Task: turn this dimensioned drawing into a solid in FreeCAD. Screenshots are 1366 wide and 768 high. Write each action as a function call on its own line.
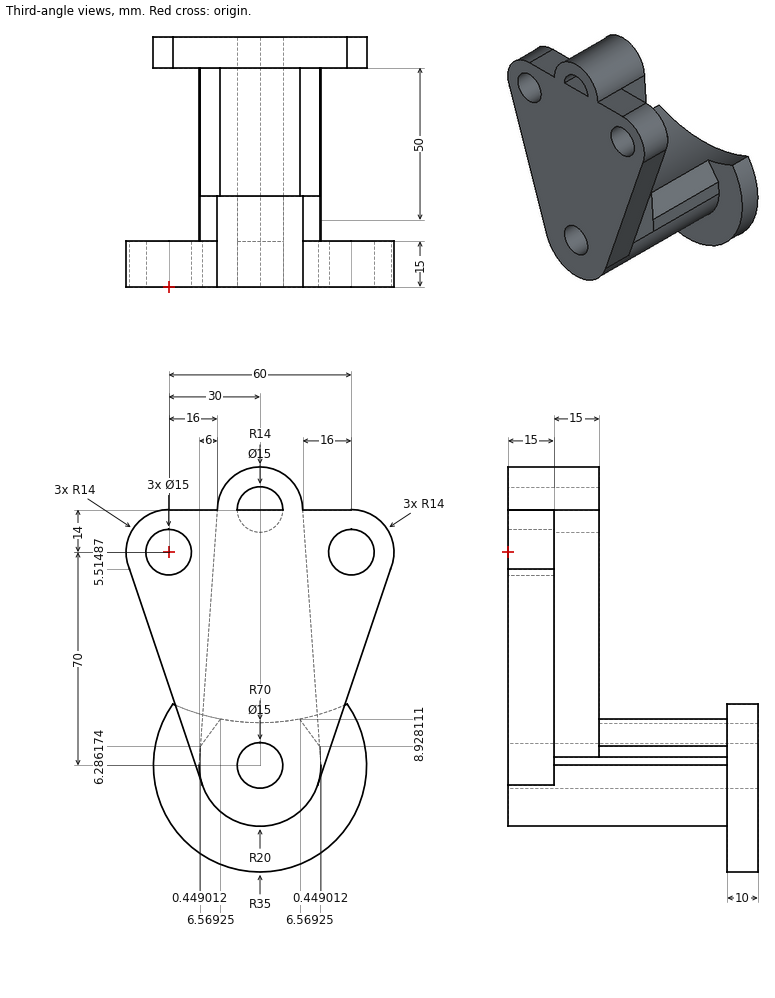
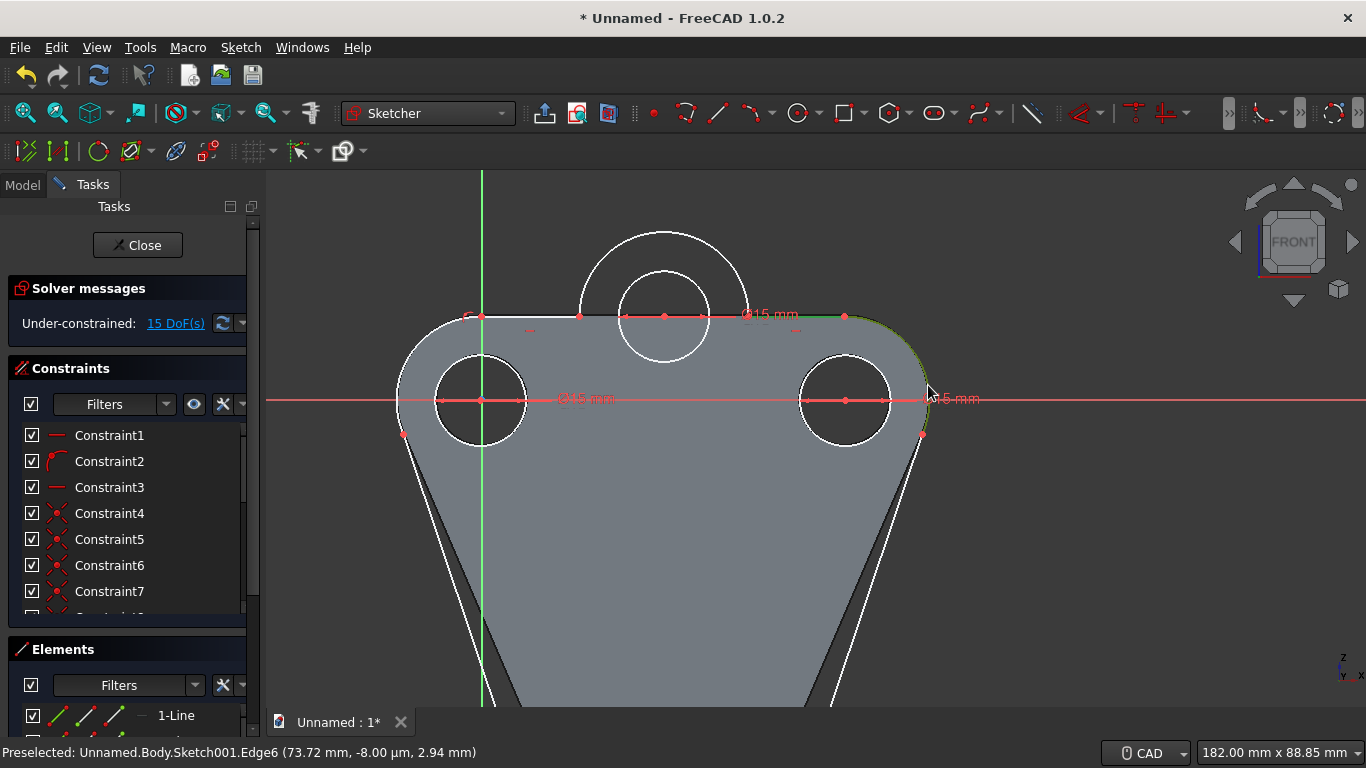
key(t)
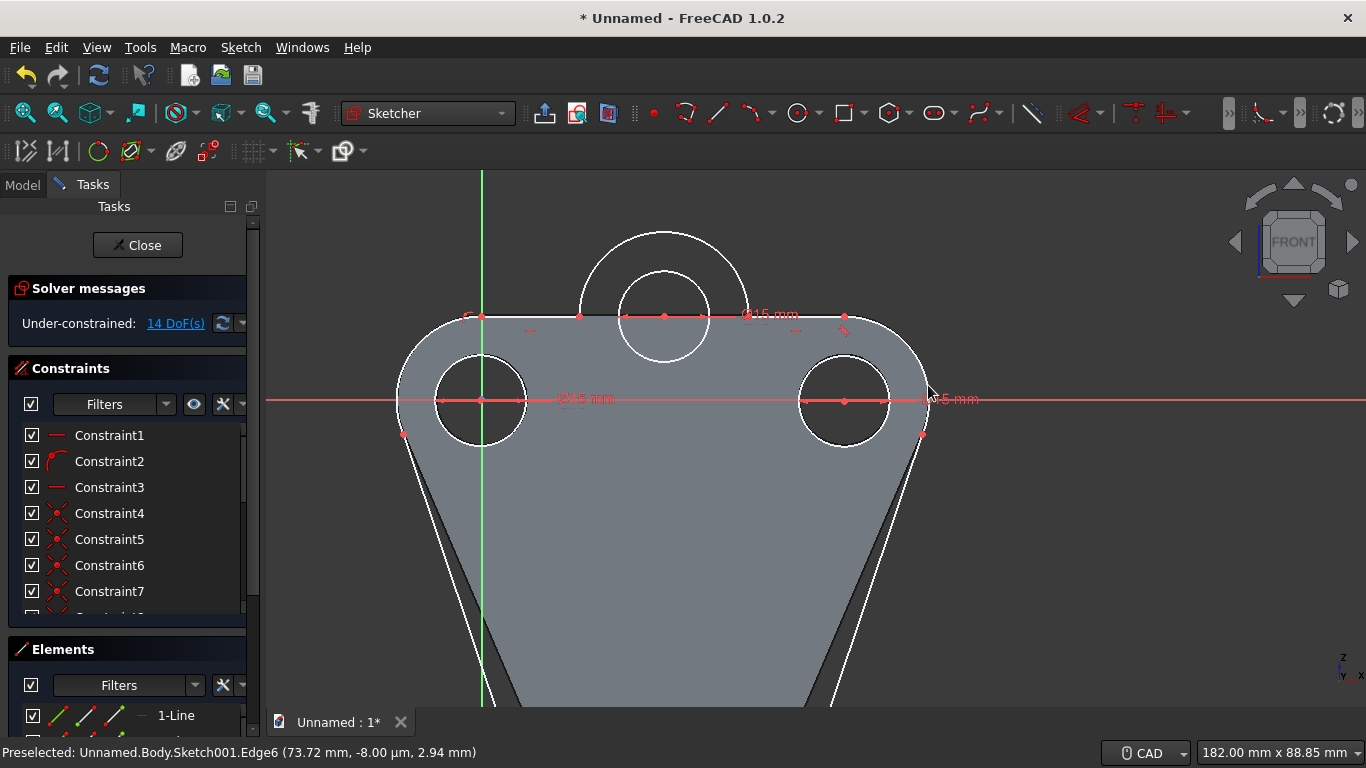
click(550, 317)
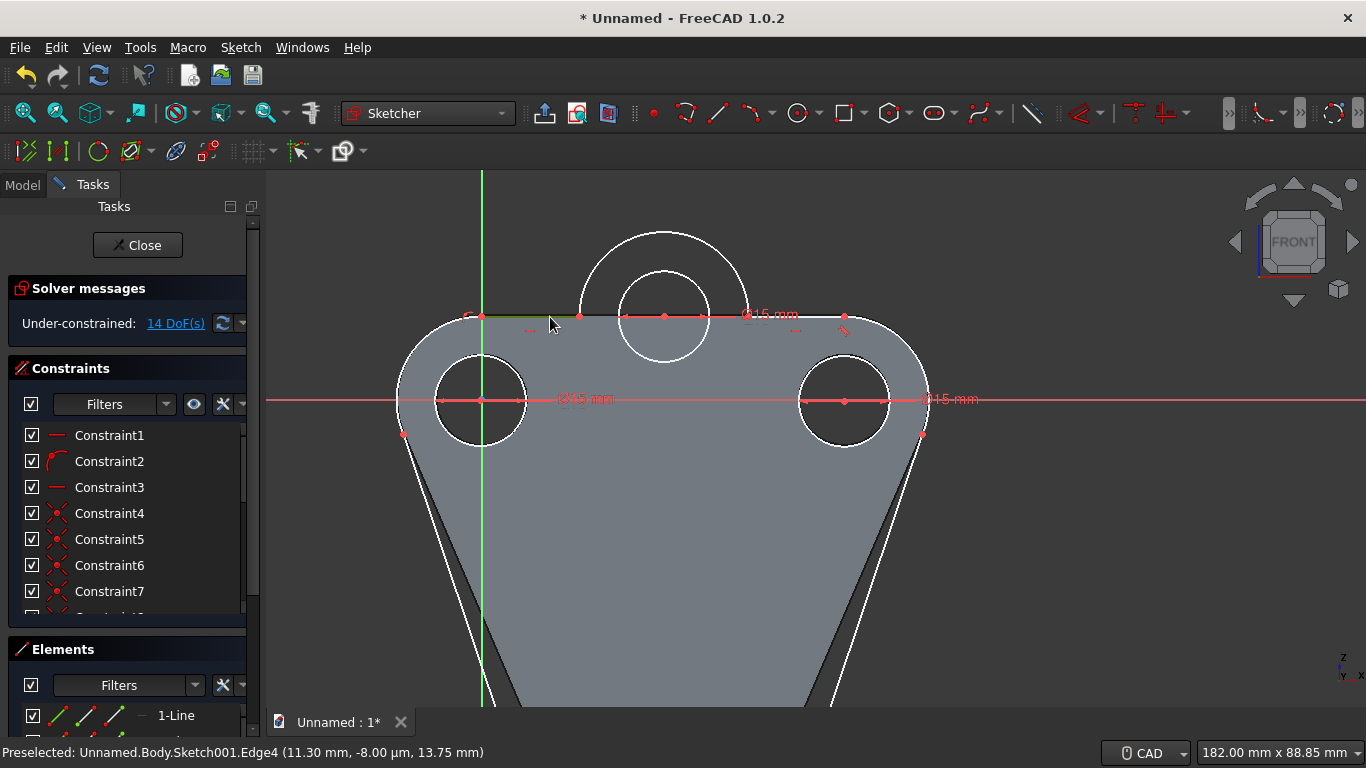
click(434, 331)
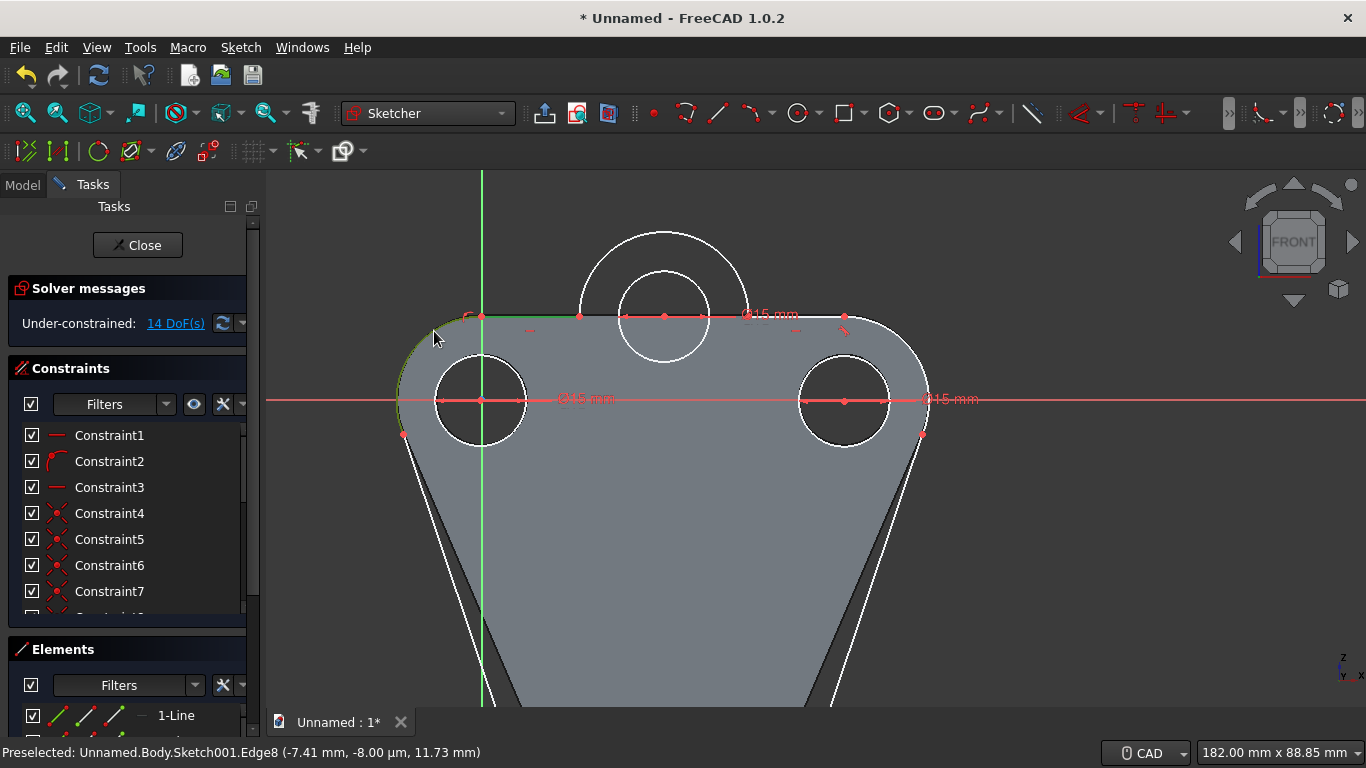
key(t)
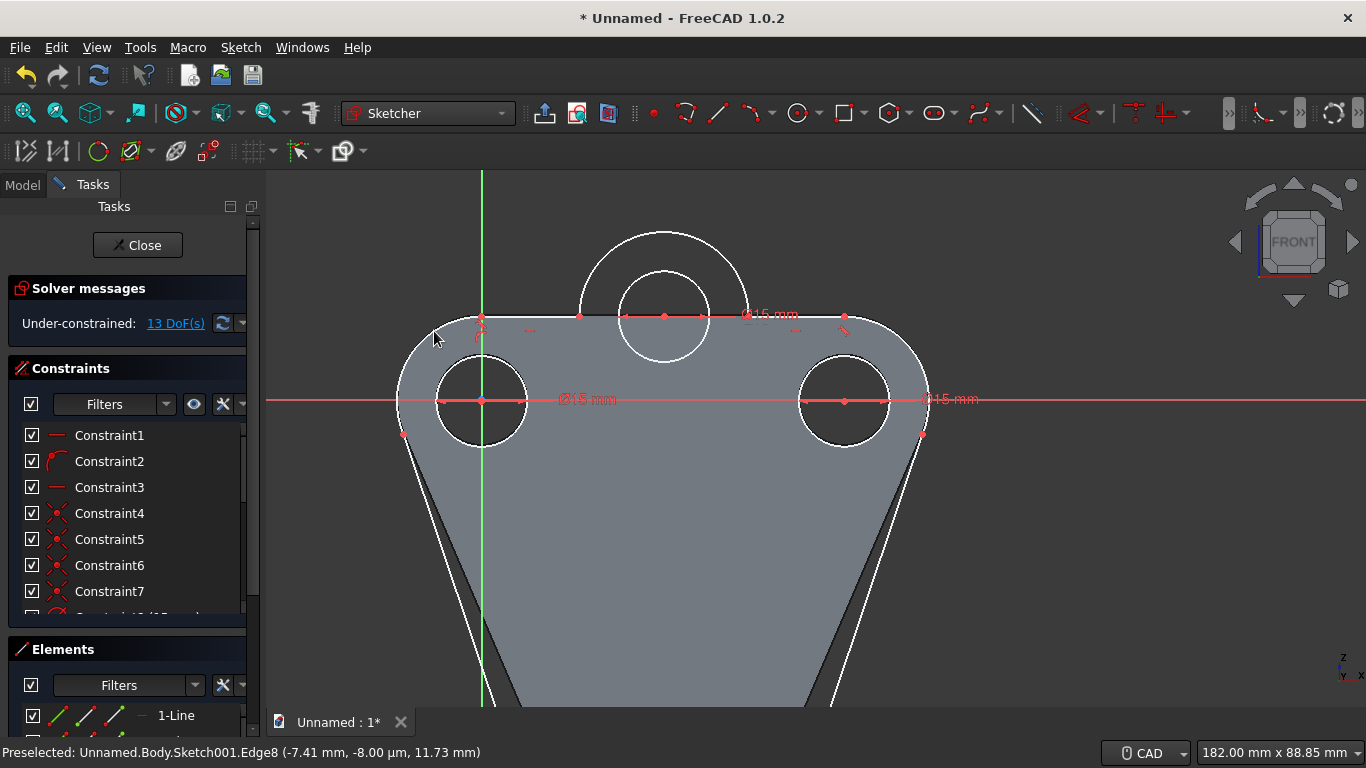
click(928, 385)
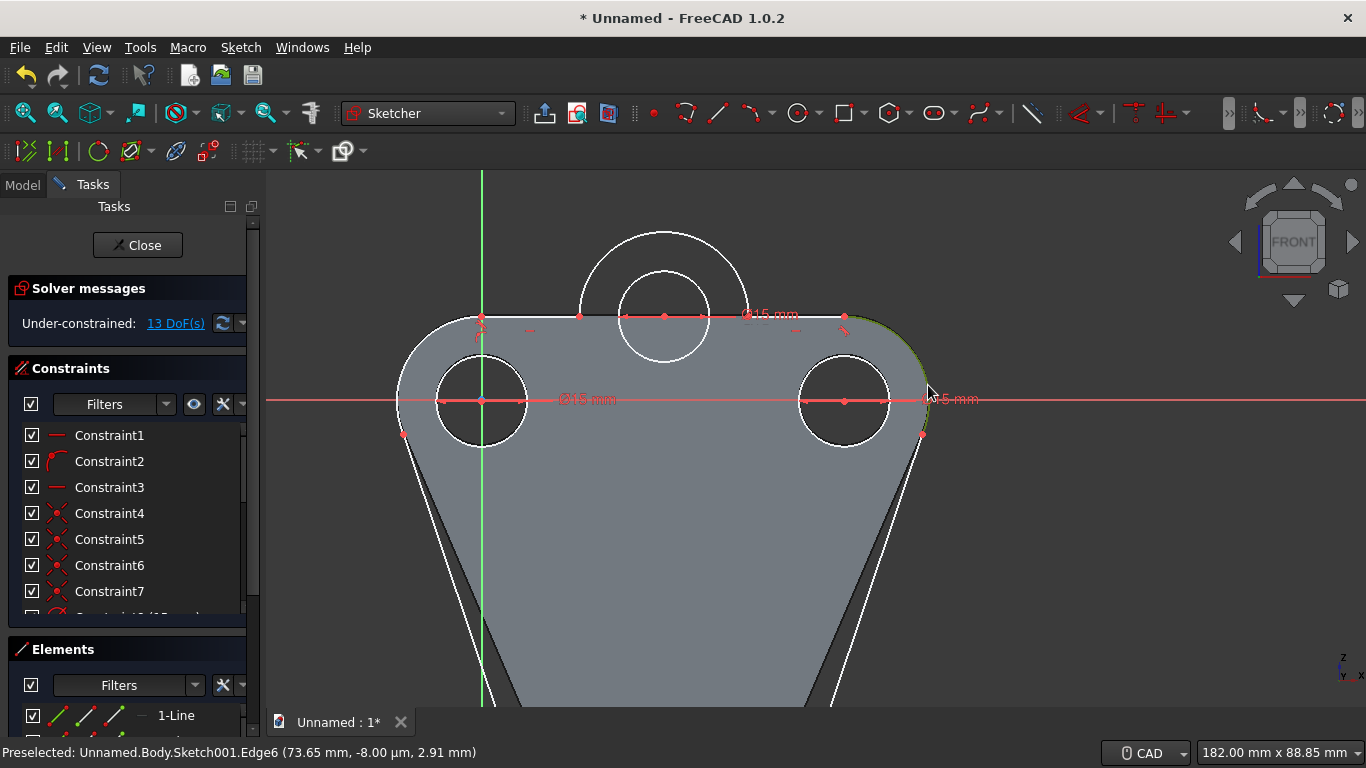
click(714, 248)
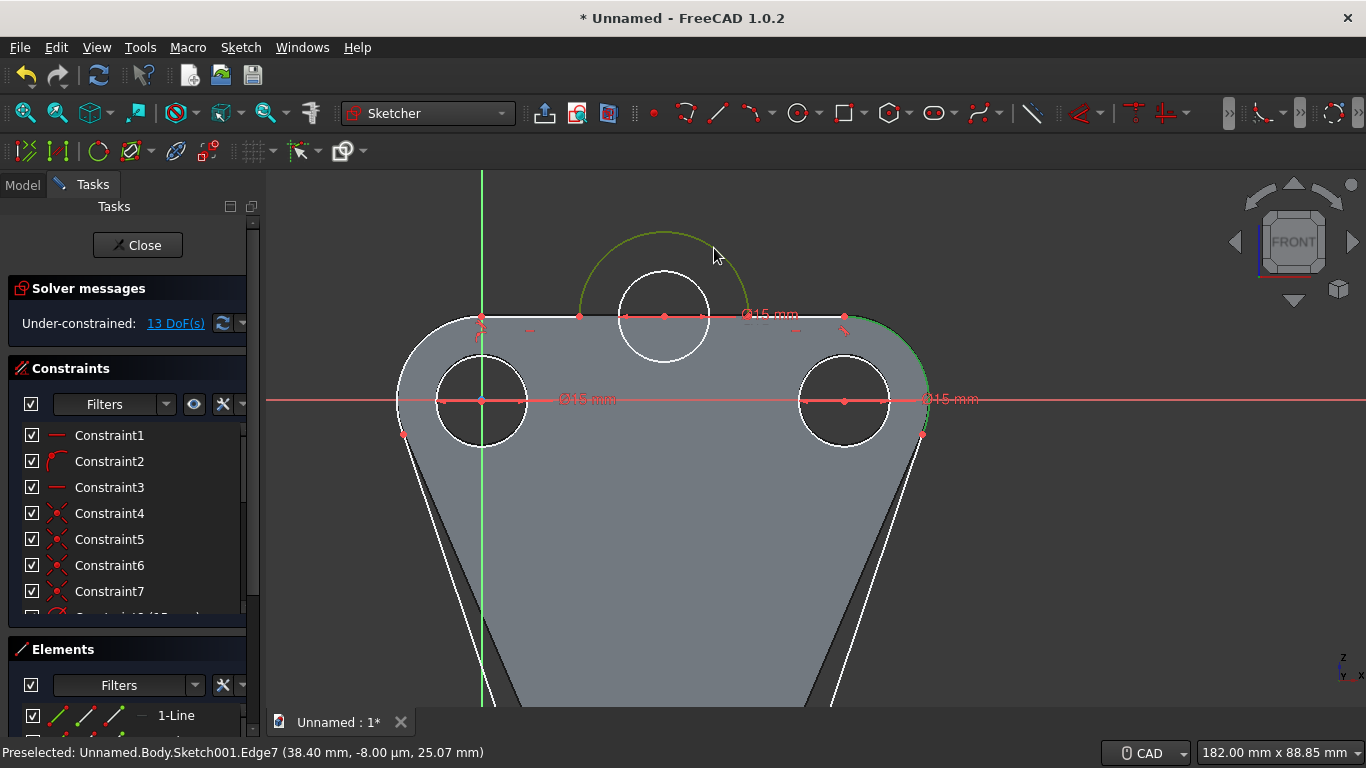
click(434, 331)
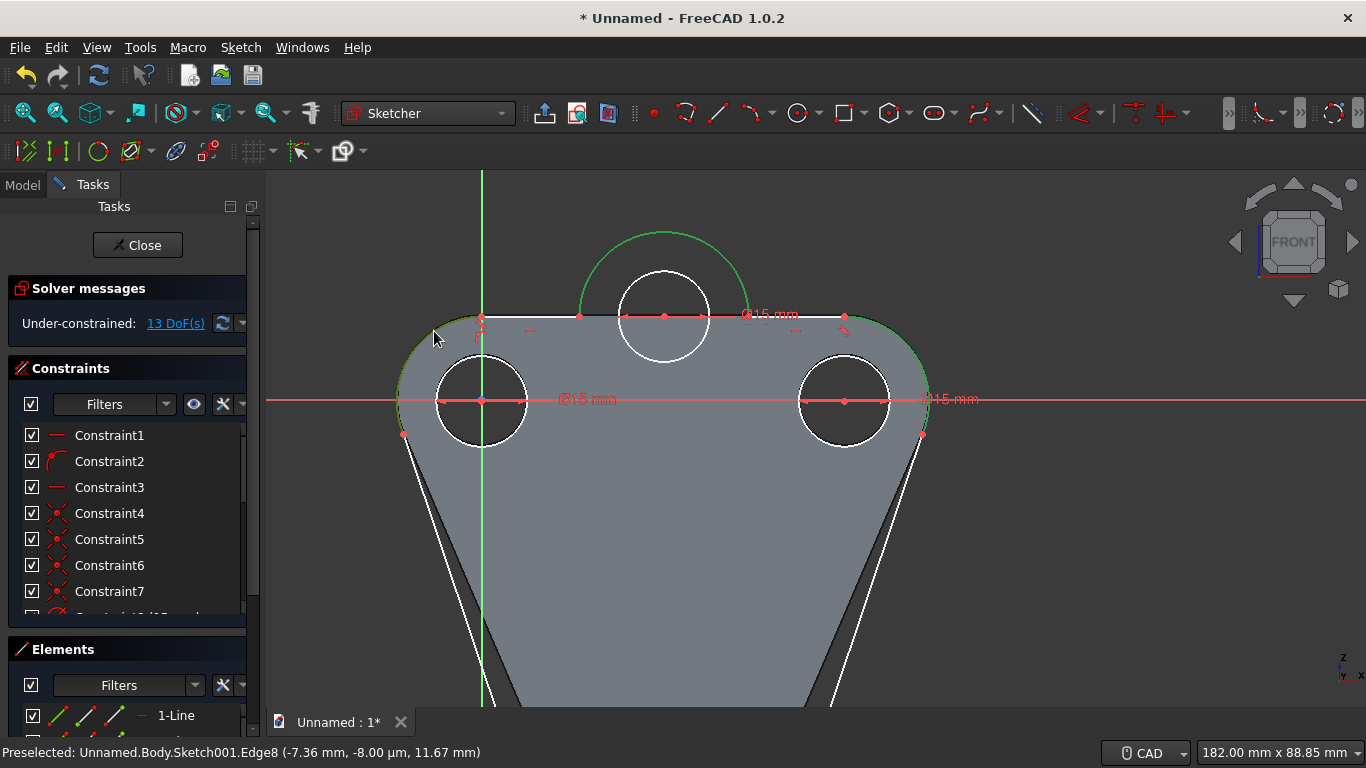
key(e)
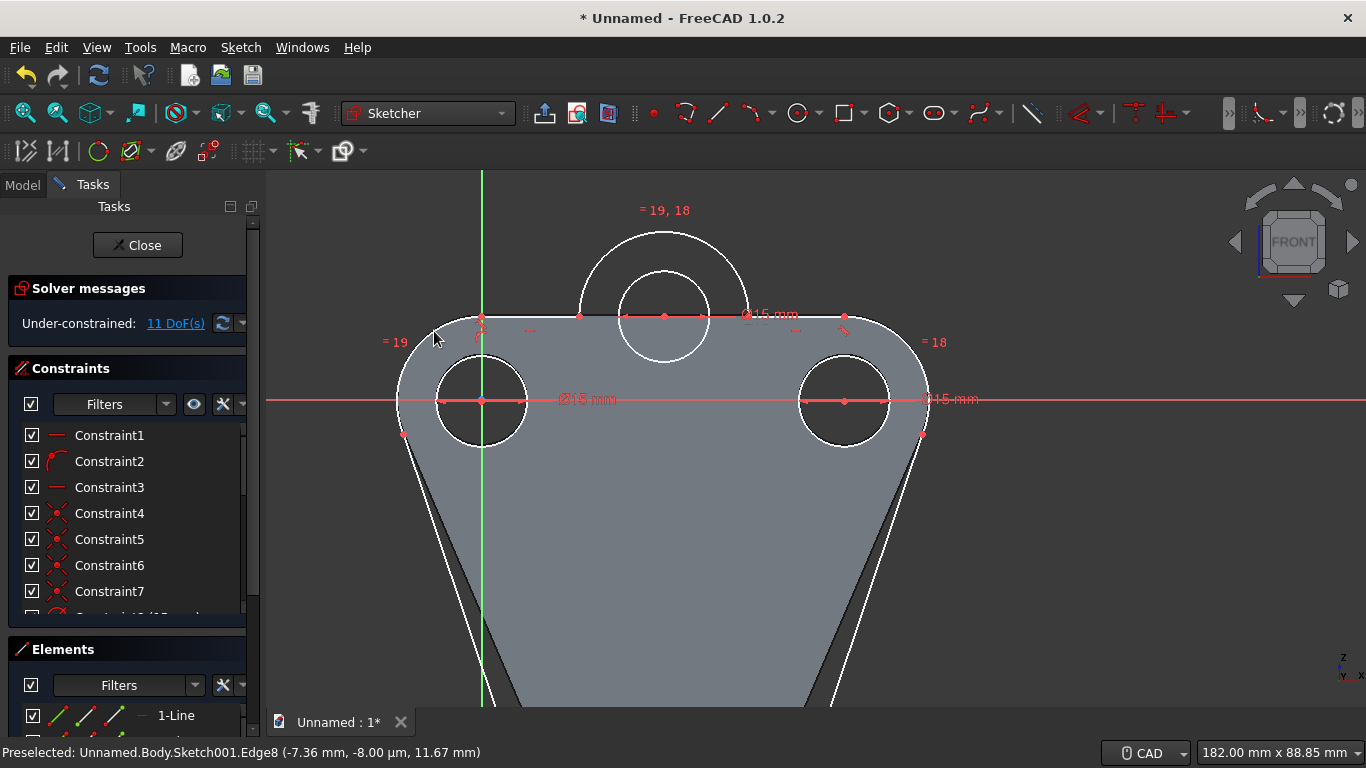
click(844, 401)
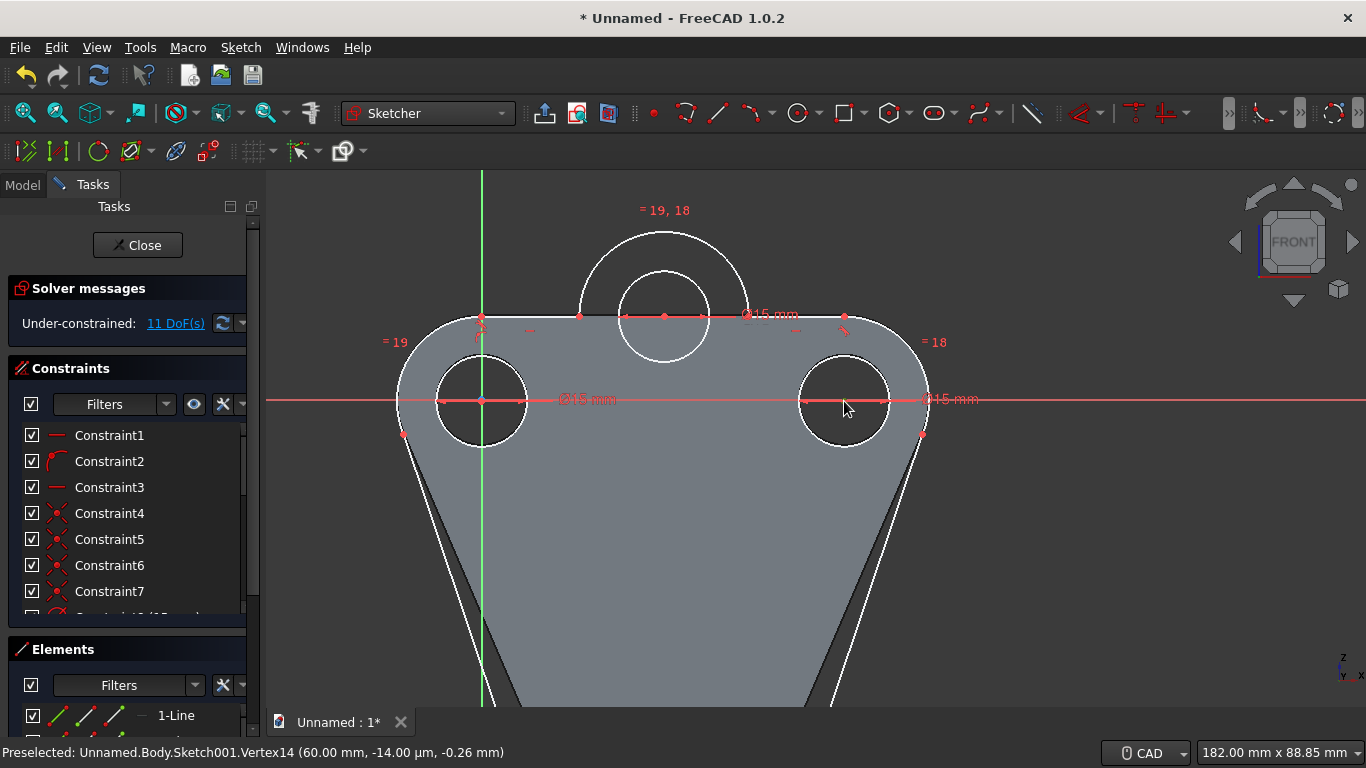
click(359, 400)